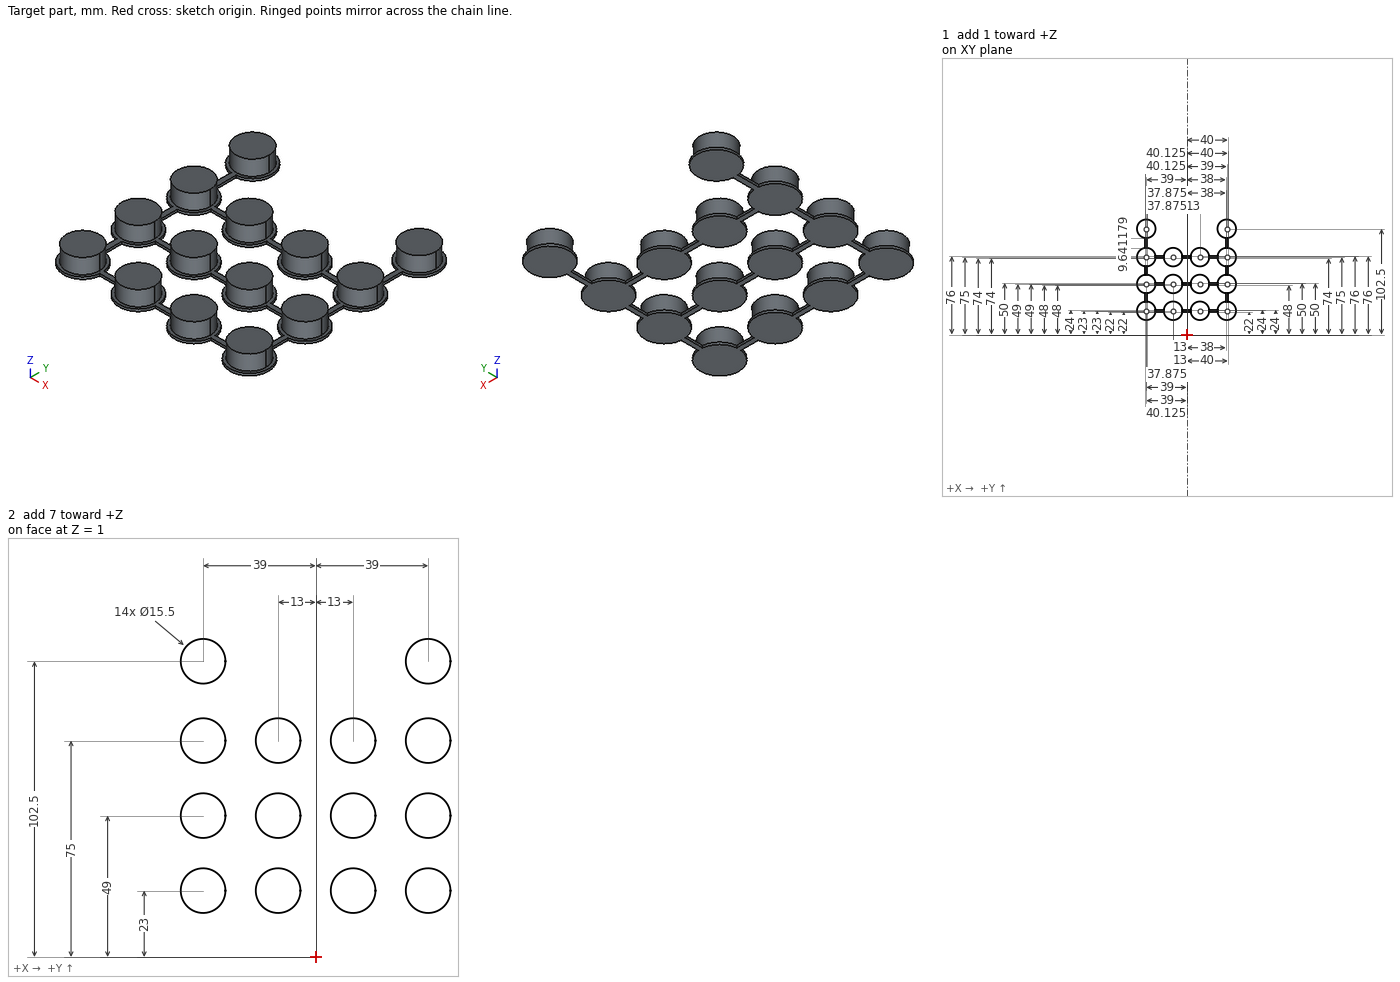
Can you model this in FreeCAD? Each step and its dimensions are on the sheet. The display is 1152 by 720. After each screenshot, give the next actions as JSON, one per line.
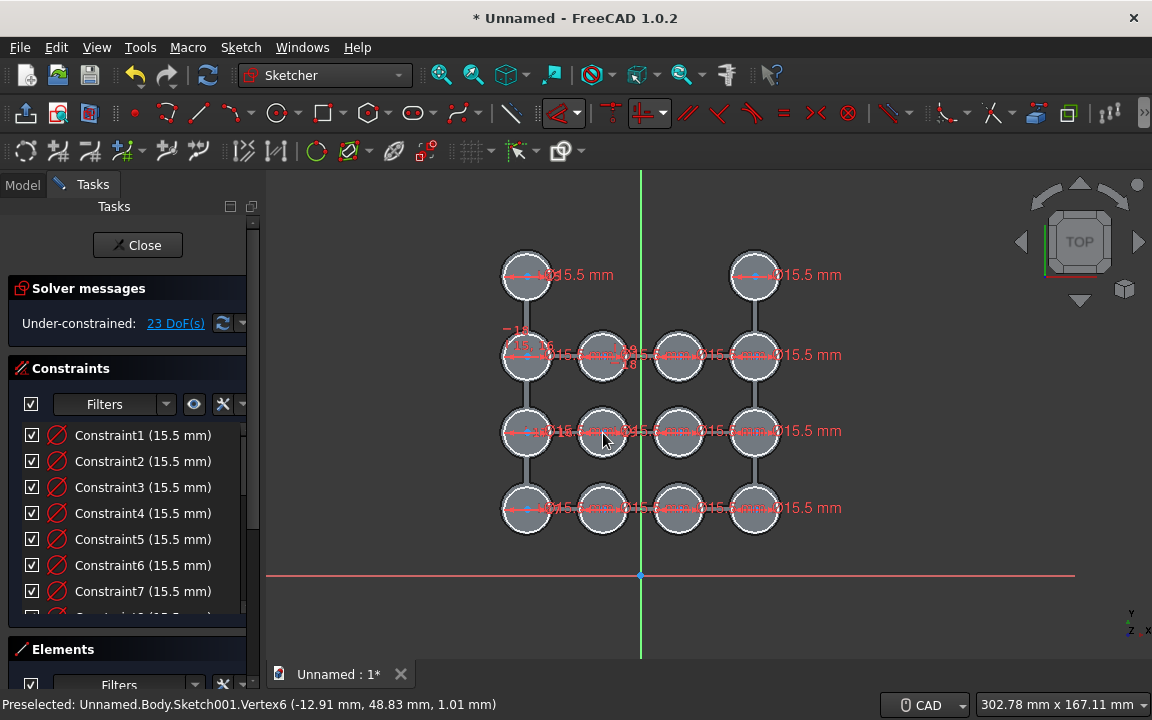
{"action": "left_click", "coordinate": [527, 433]}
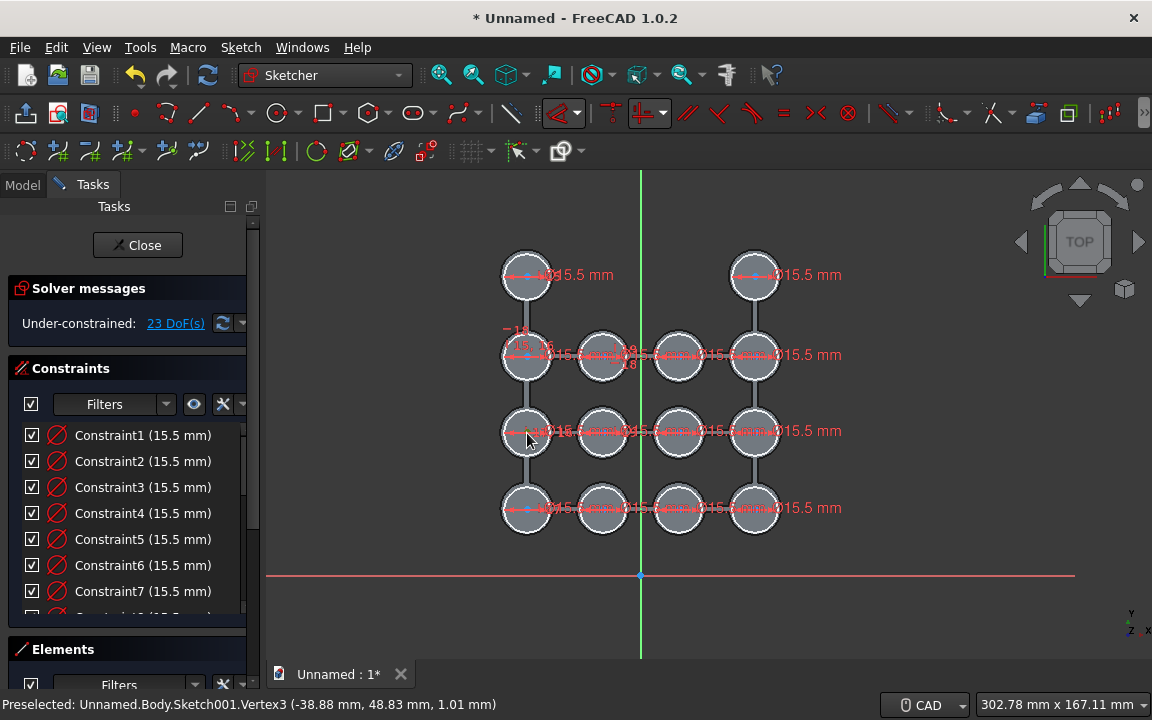
{"action": "left_click", "coordinate": [603, 433]}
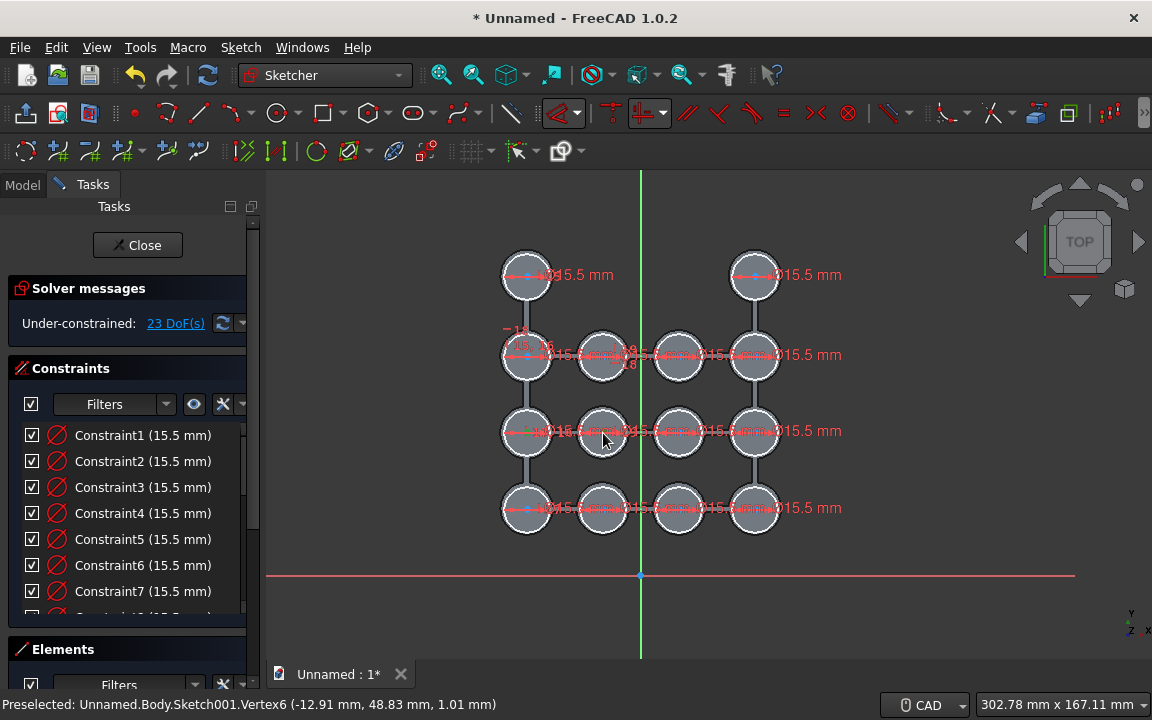
{"action": "left_click", "coordinate": [666, 114]}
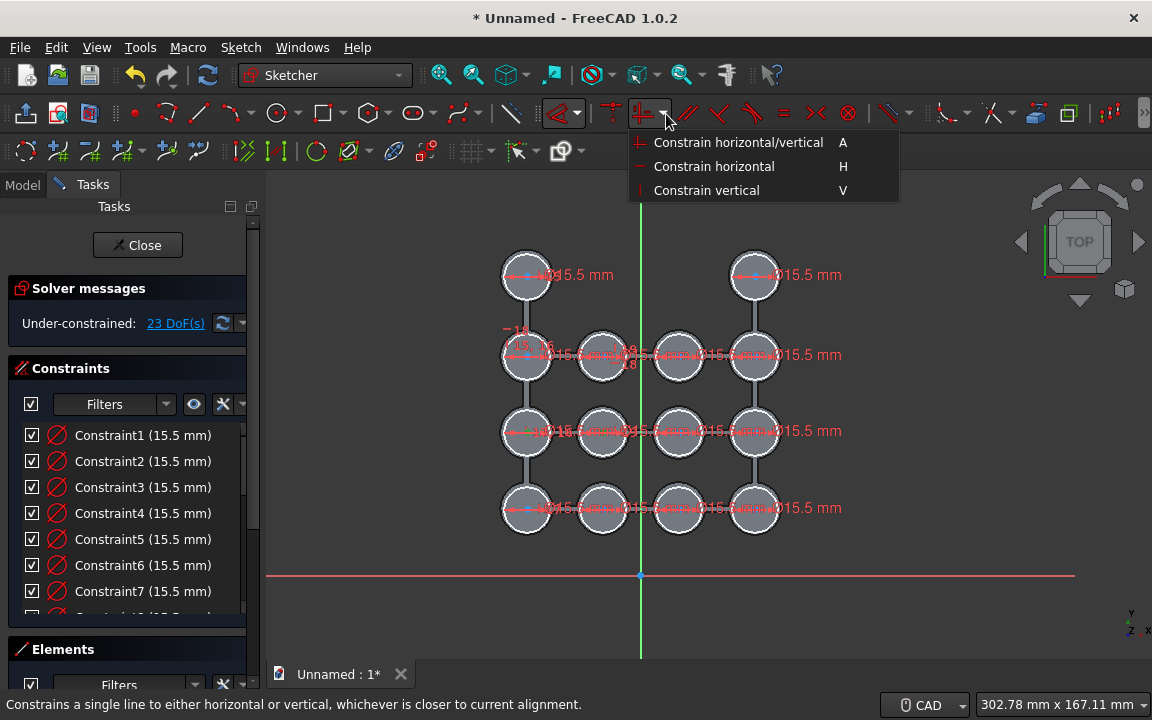
{"action": "left_click", "coordinate": [764, 166]}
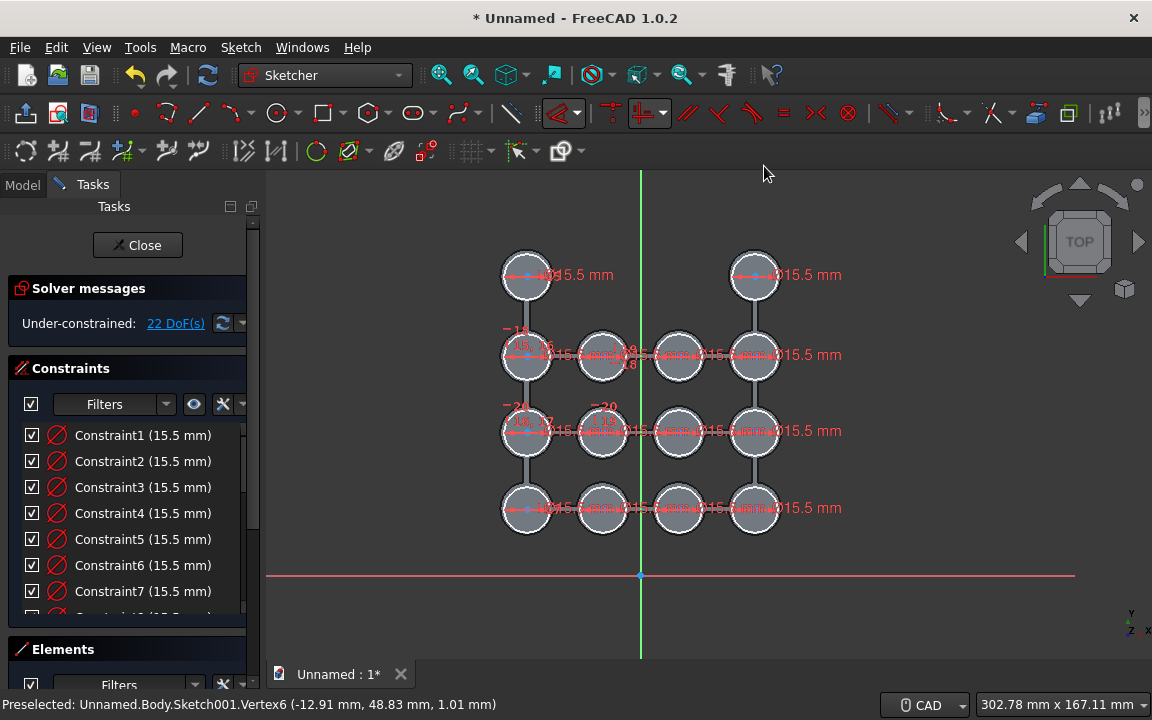
{"action": "left_click", "coordinate": [603, 433]}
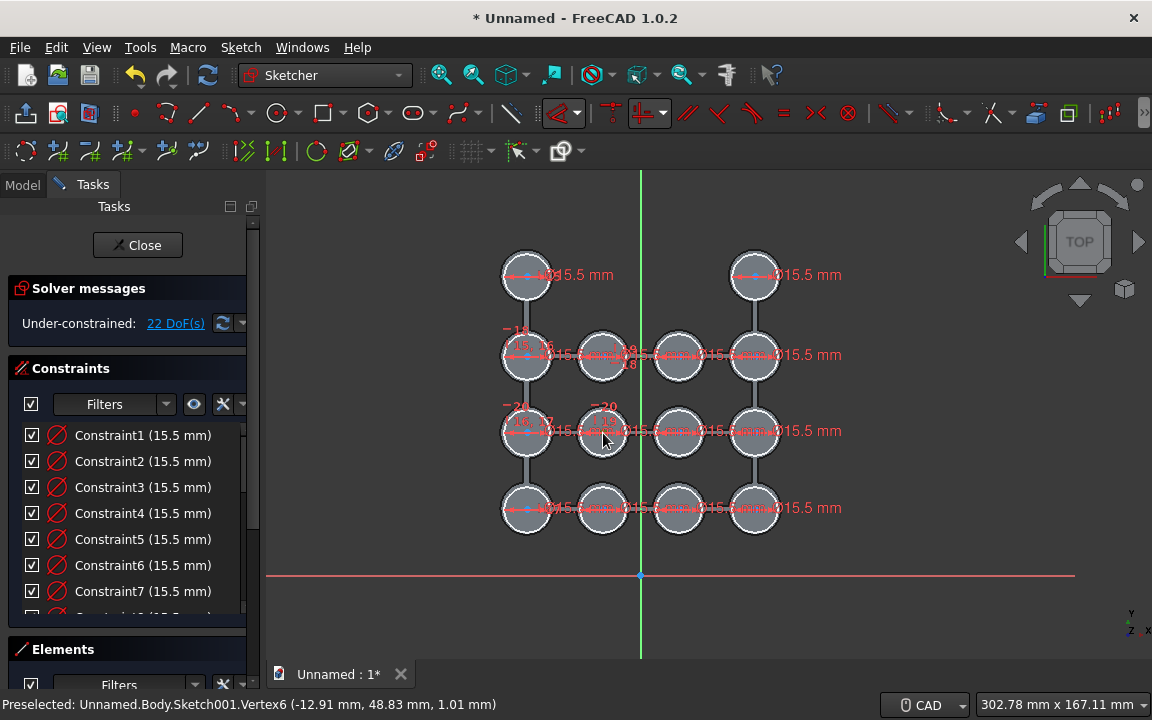
{"action": "left_click", "coordinate": [603, 510]}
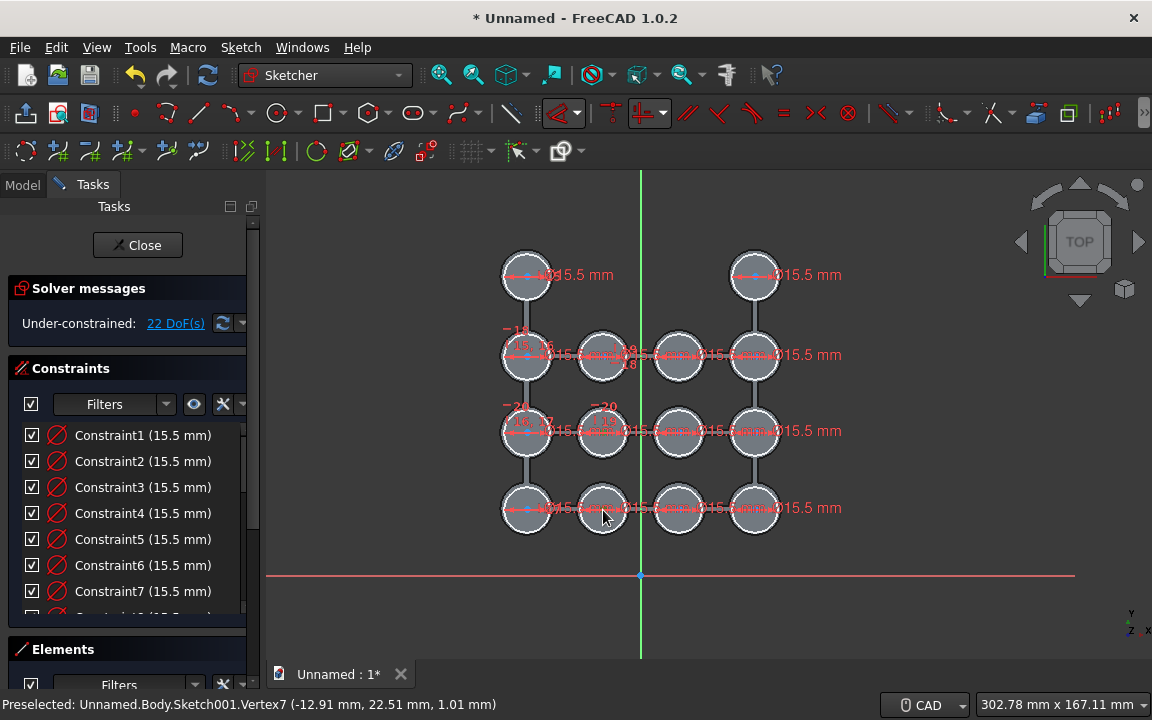
{"action": "left_click", "coordinate": [666, 114]}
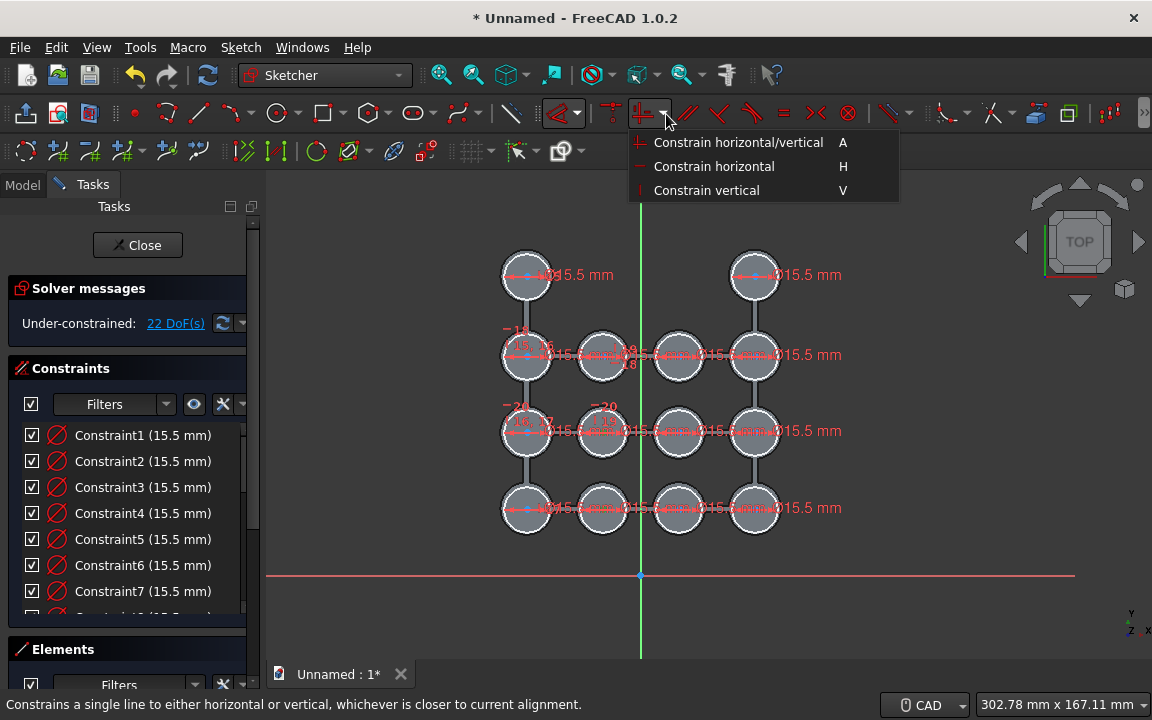
{"action": "left_click", "coordinate": [764, 190]}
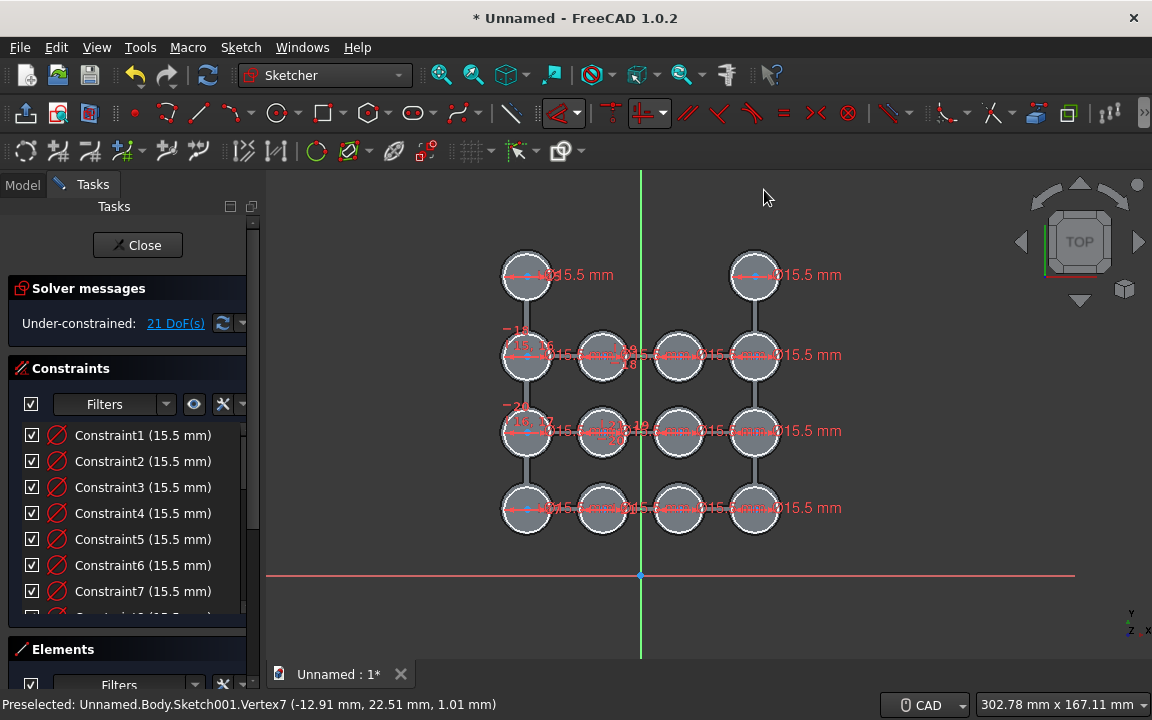
{"action": "left_click", "coordinate": [527, 510]}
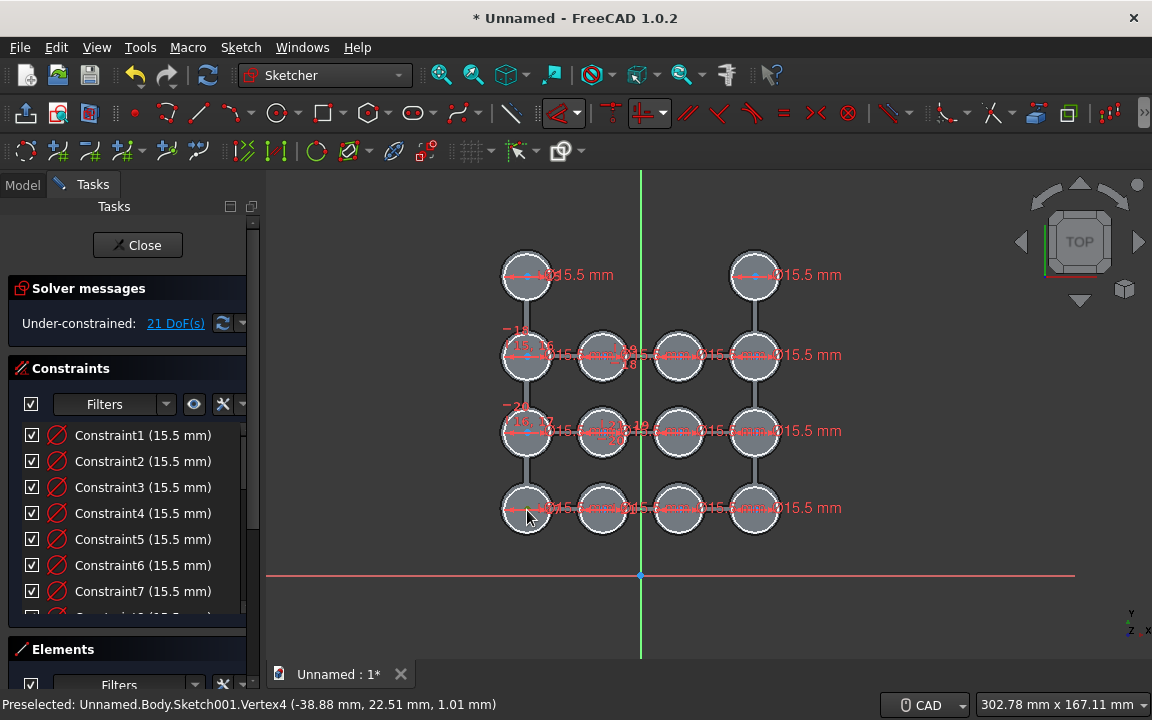
{"action": "left_click", "coordinate": [603, 510]}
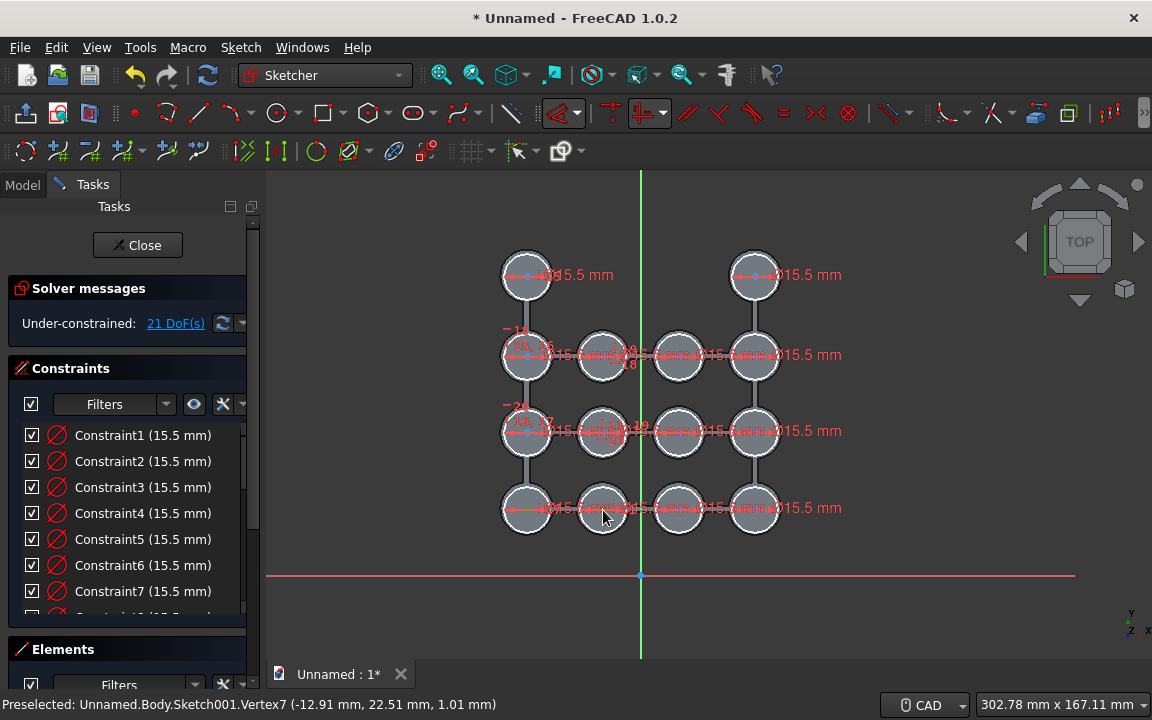
{"action": "key", "text": "h"}